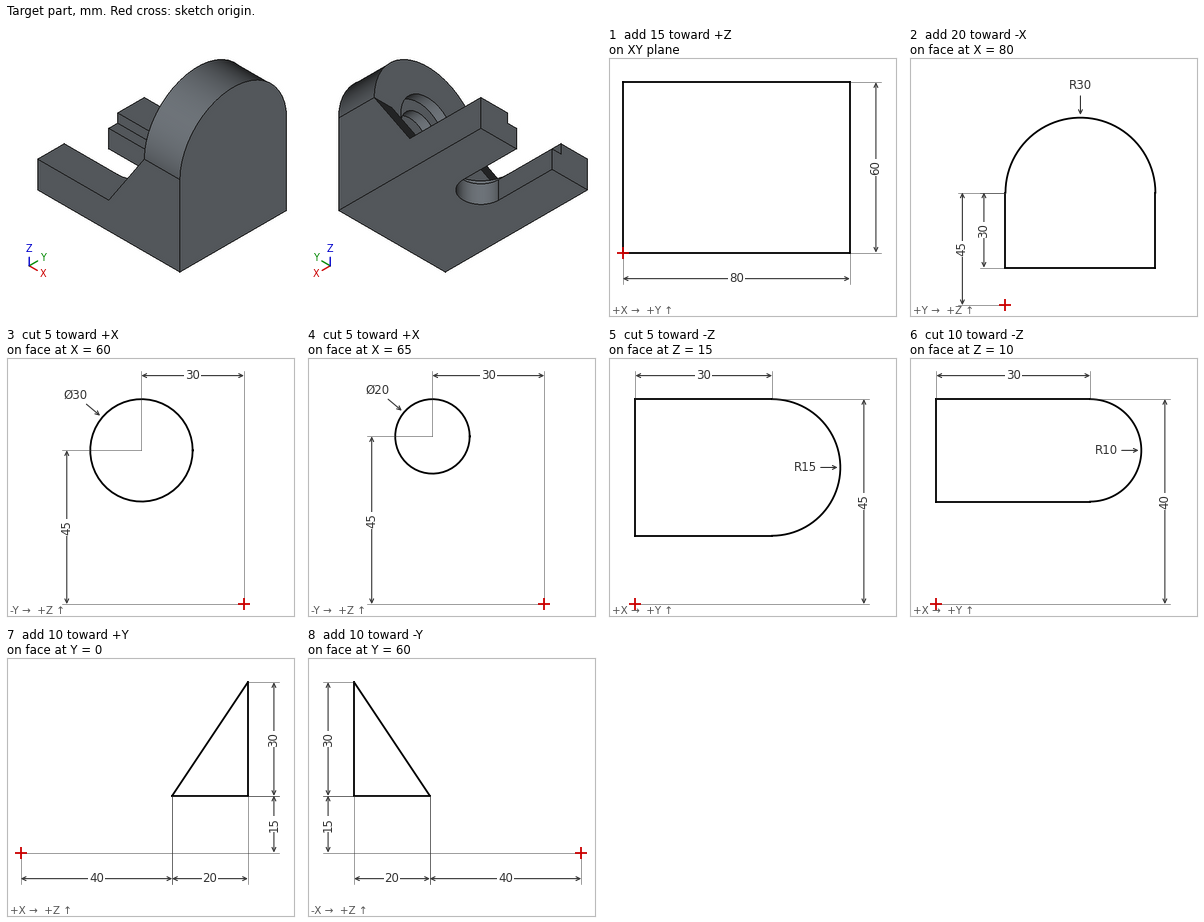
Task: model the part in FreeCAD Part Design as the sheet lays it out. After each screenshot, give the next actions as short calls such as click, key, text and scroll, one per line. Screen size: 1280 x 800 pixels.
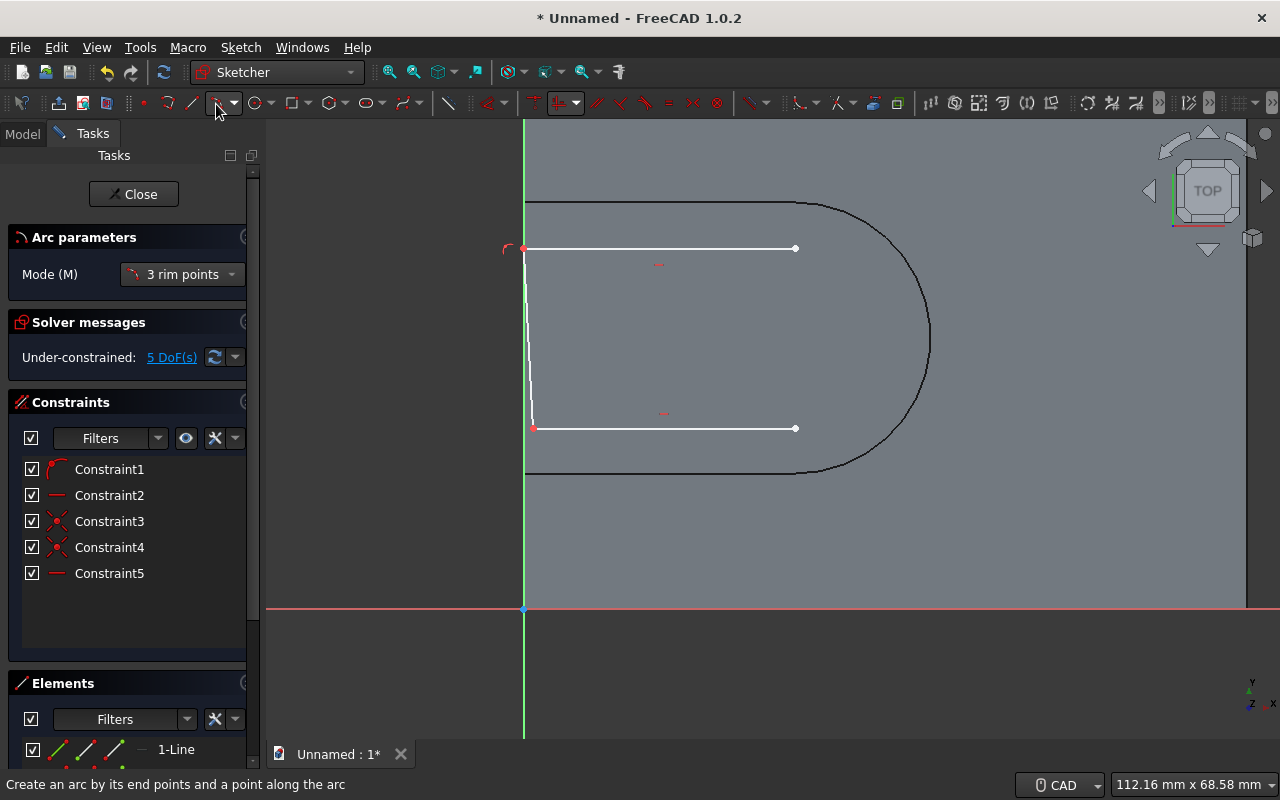
click(795, 429)
click(795, 249)
click(885, 338)
key(Escape)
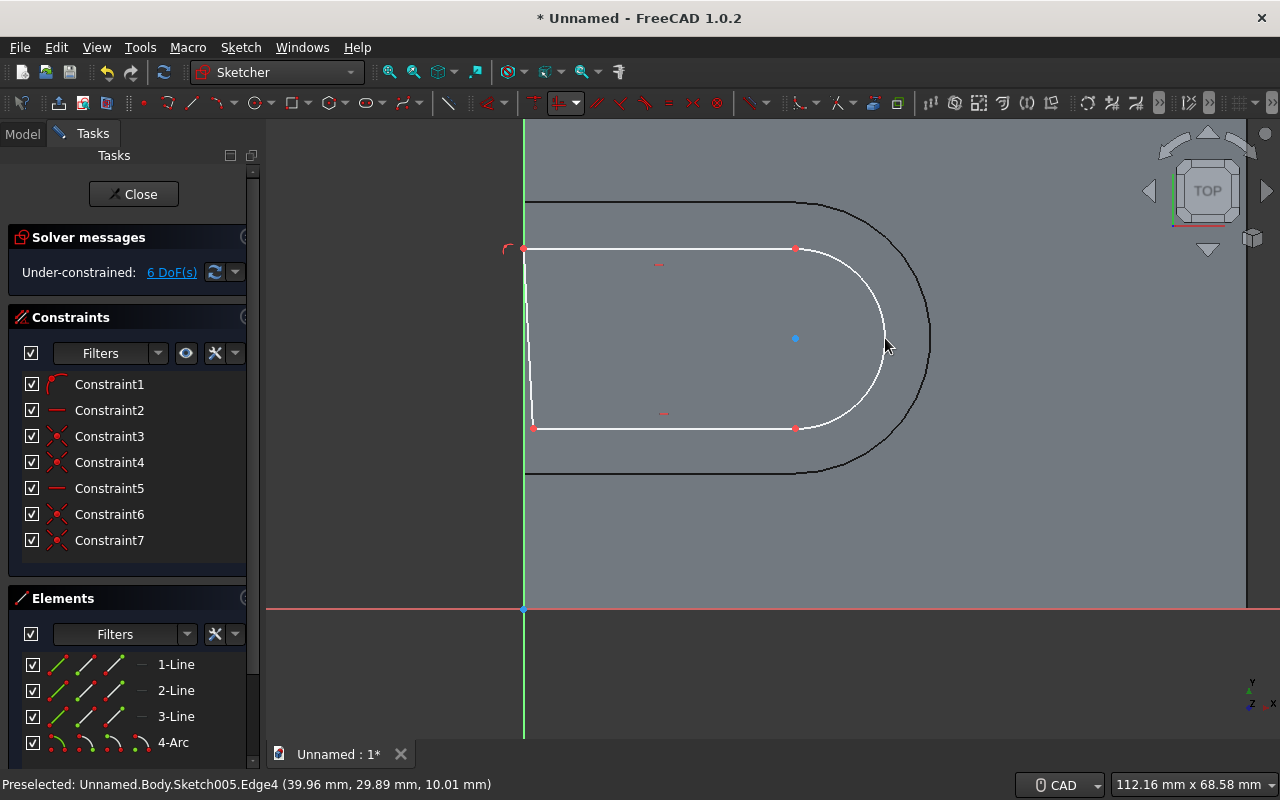
click(714, 249)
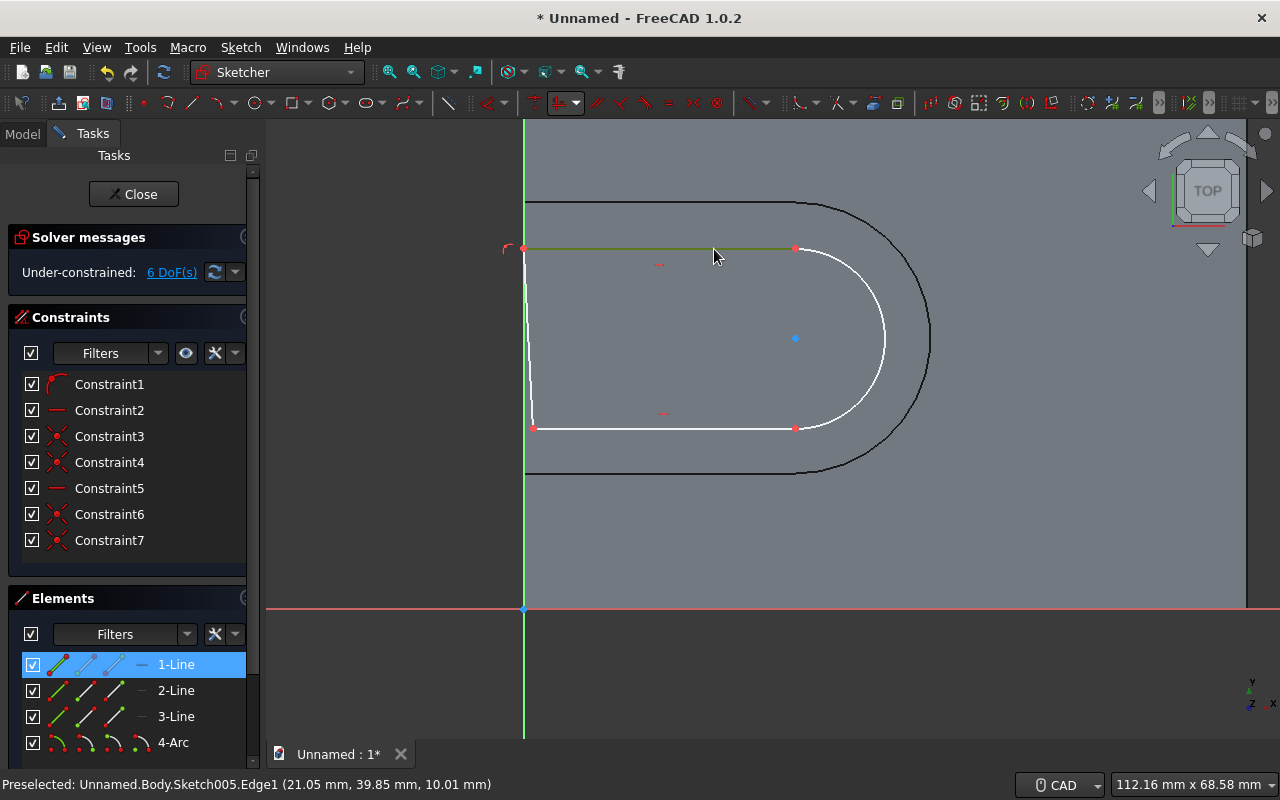
click(868, 392)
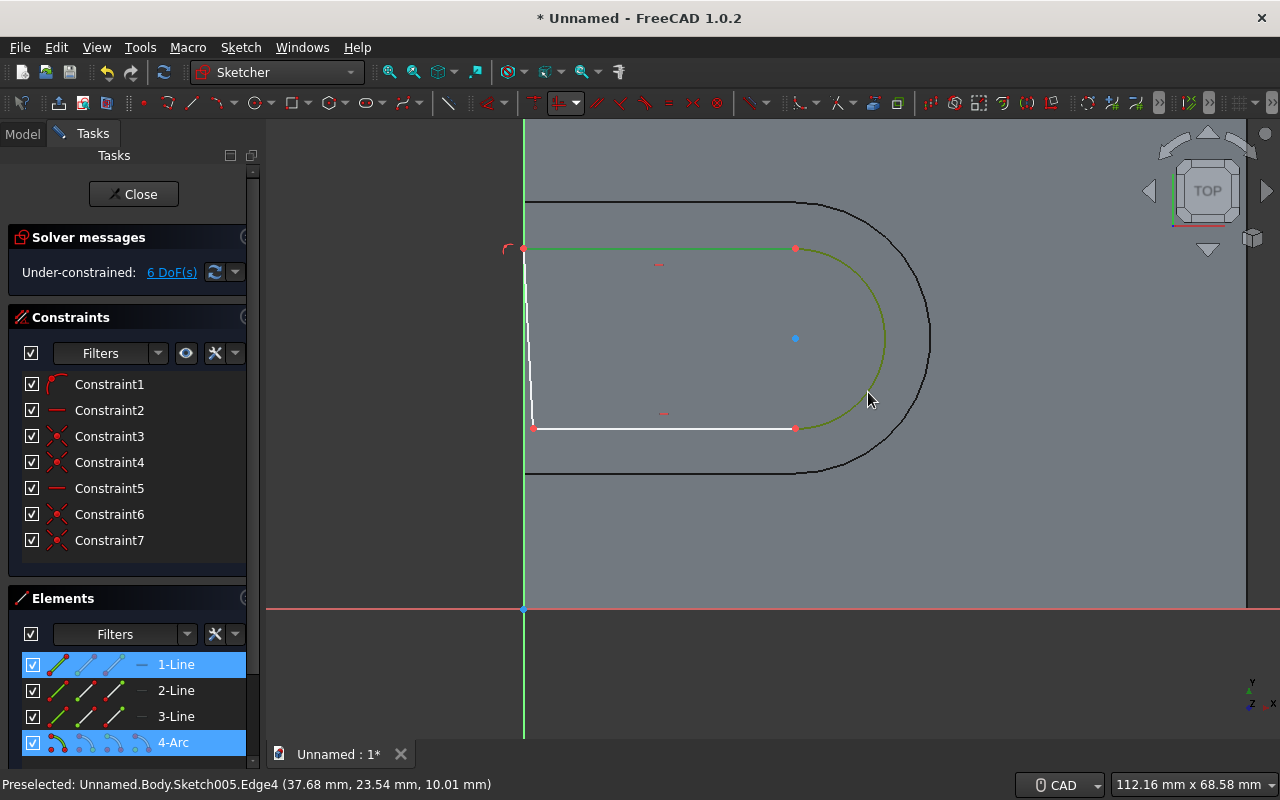
click(646, 104)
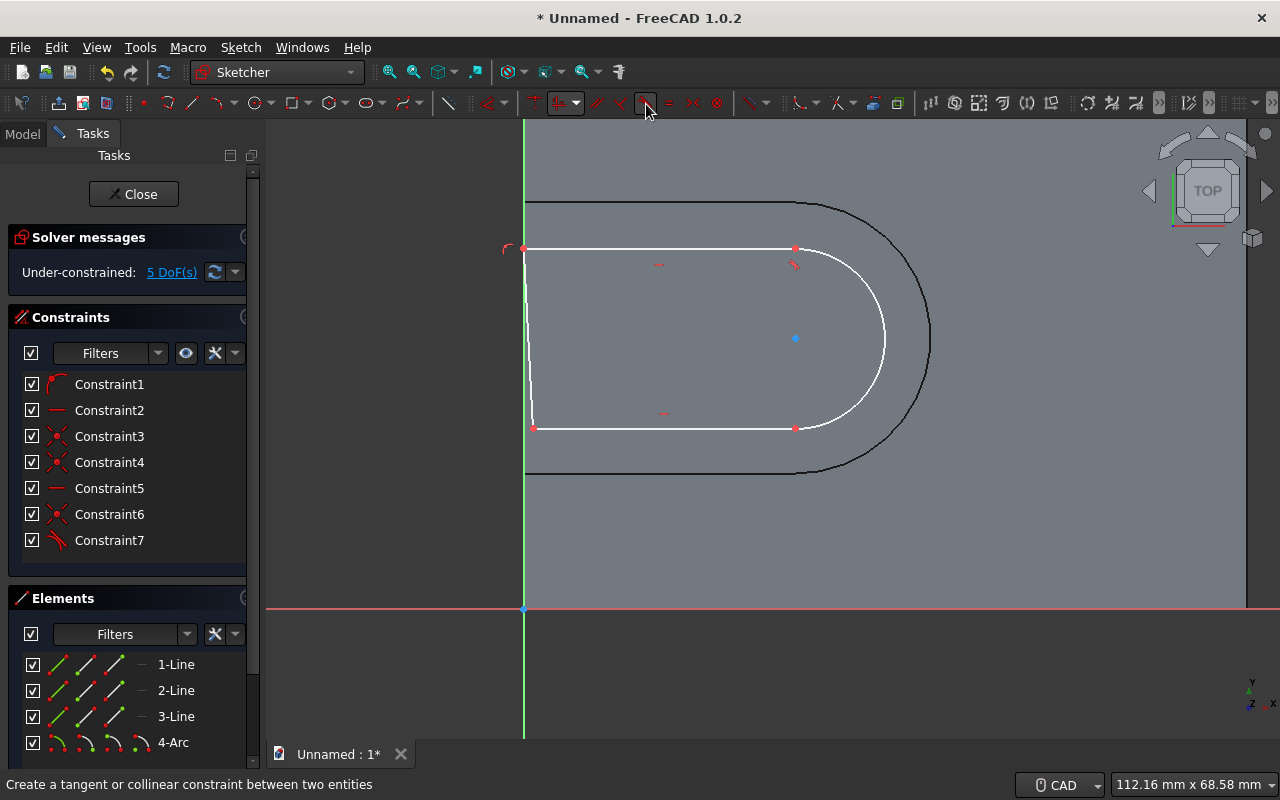
click(612, 429)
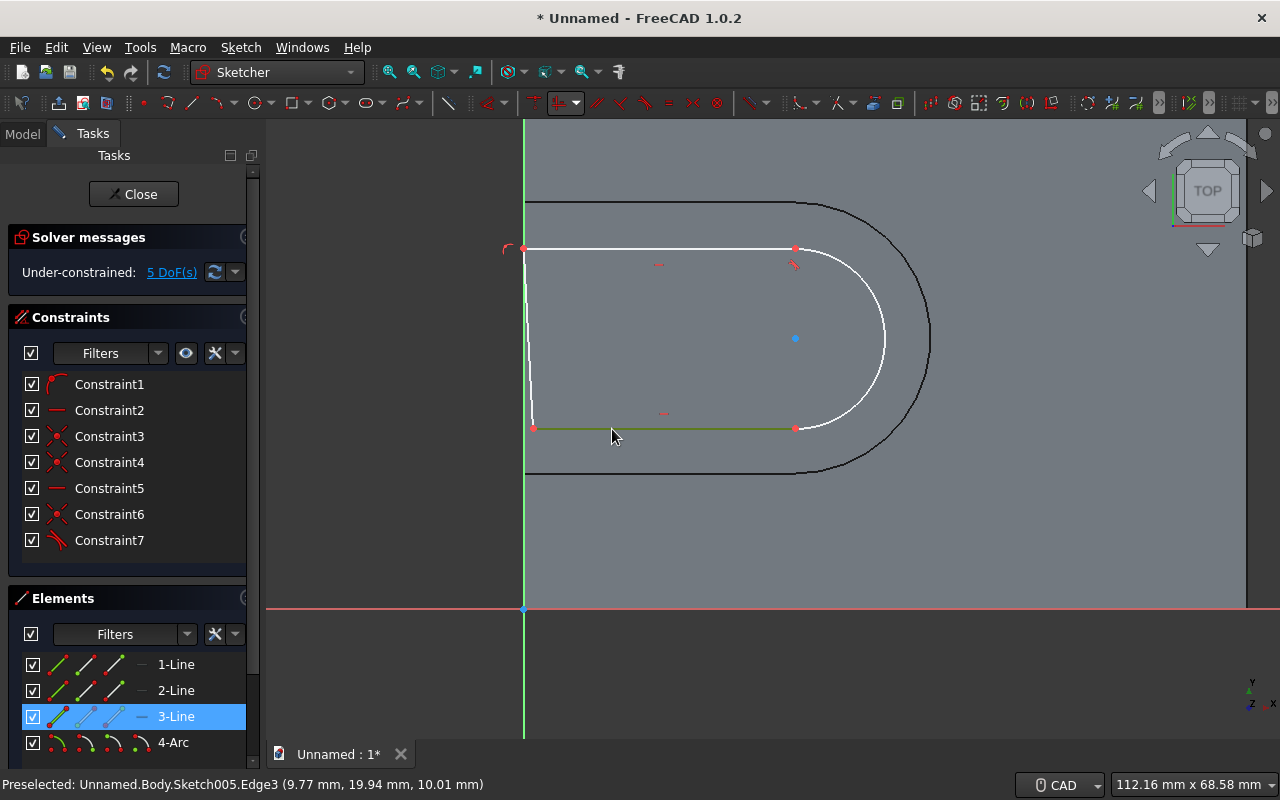
click(868, 392)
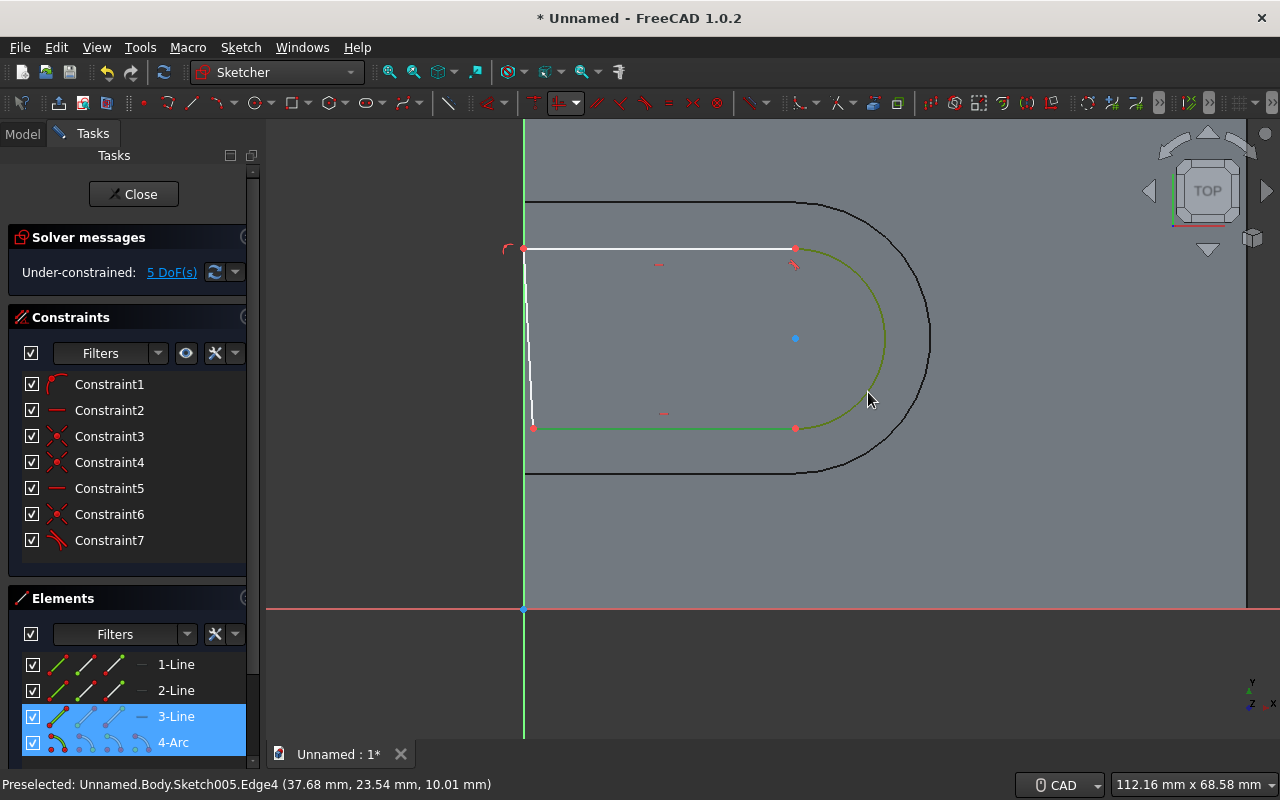
click(646, 104)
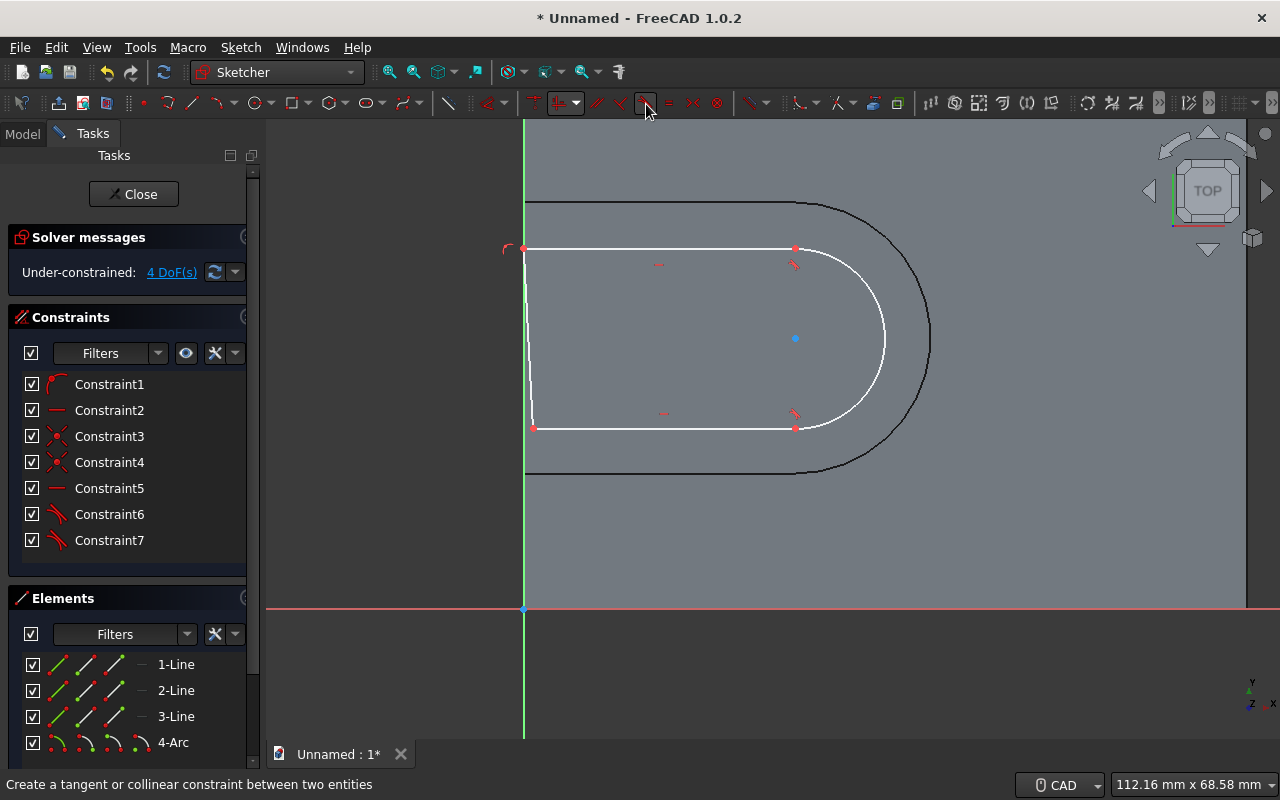
click(526, 303)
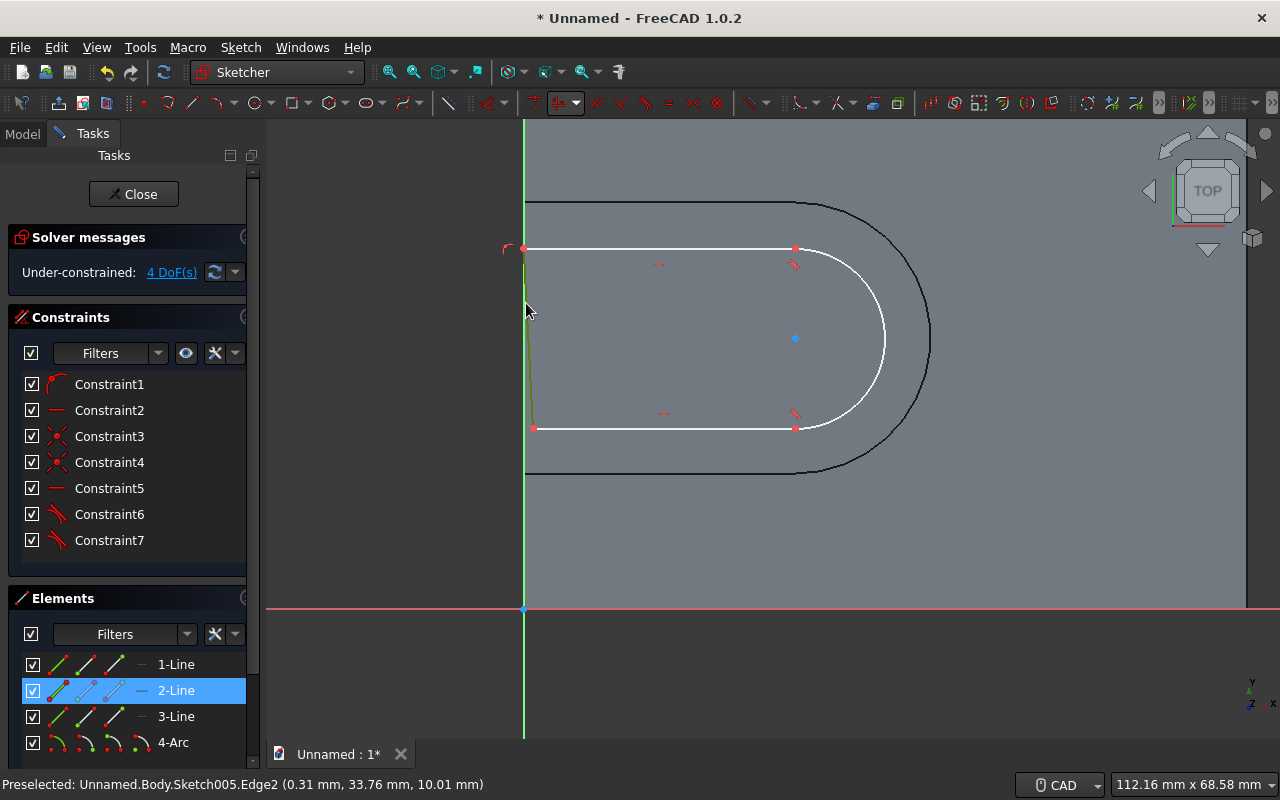
key(v)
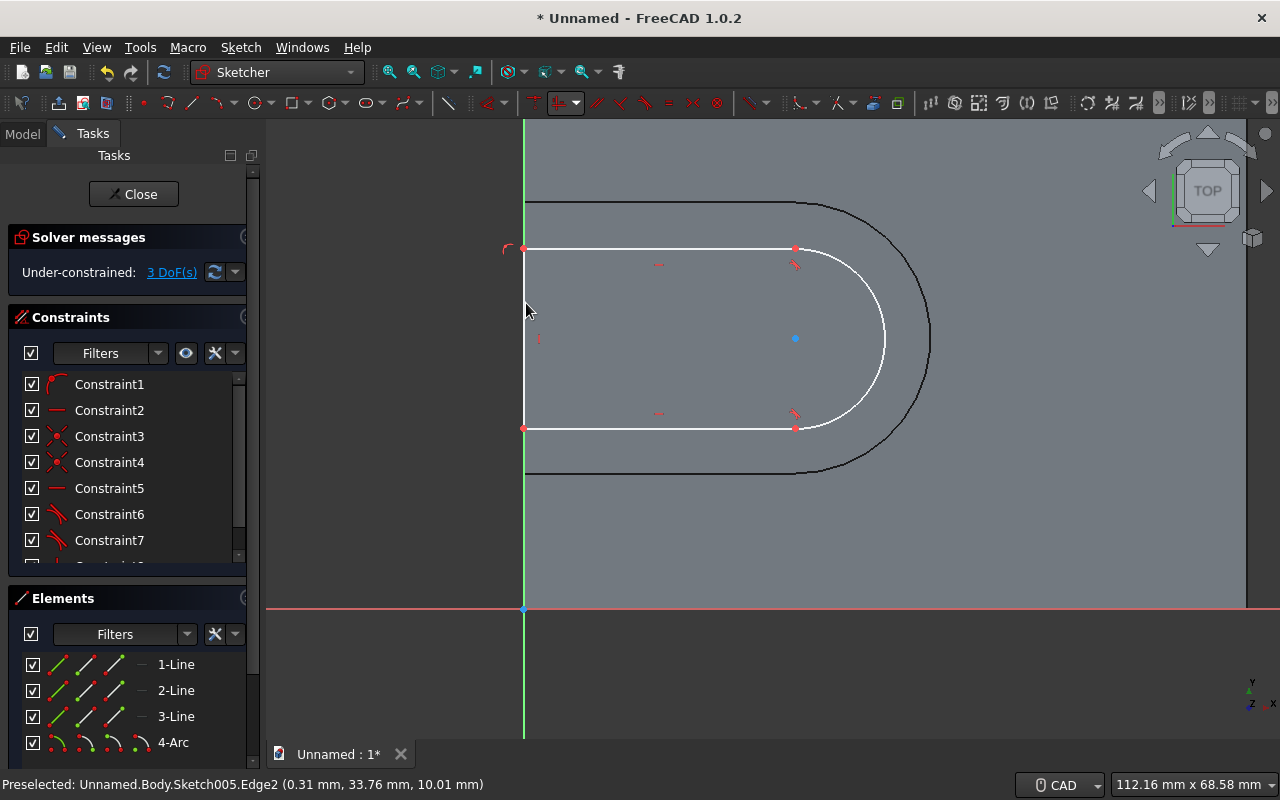
click(488, 104)